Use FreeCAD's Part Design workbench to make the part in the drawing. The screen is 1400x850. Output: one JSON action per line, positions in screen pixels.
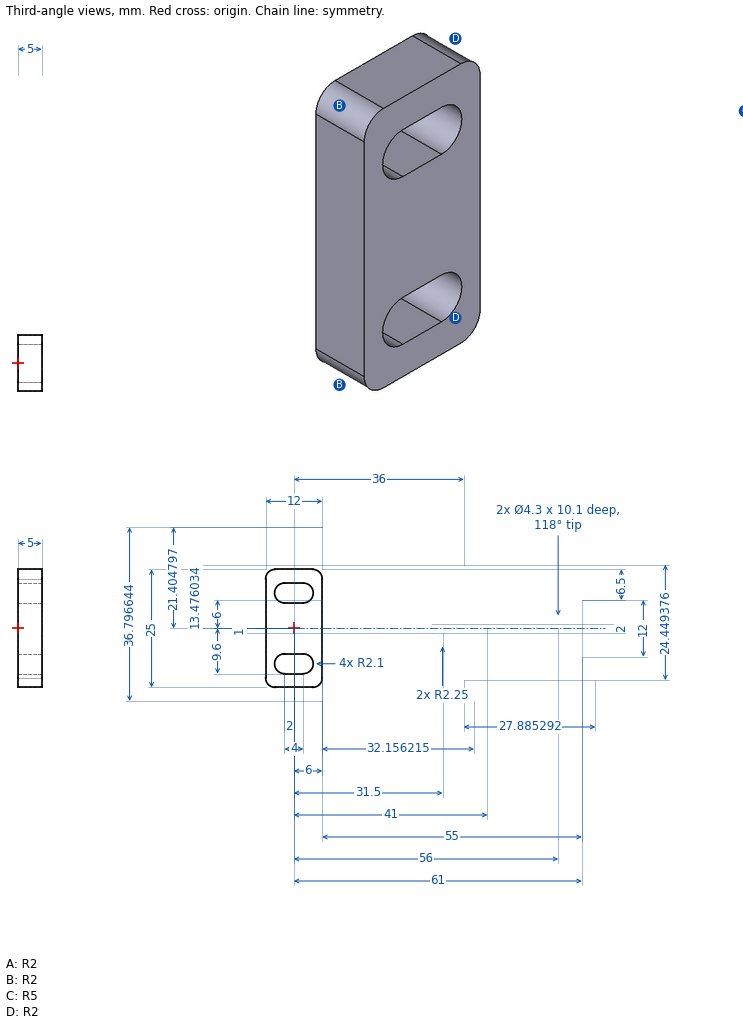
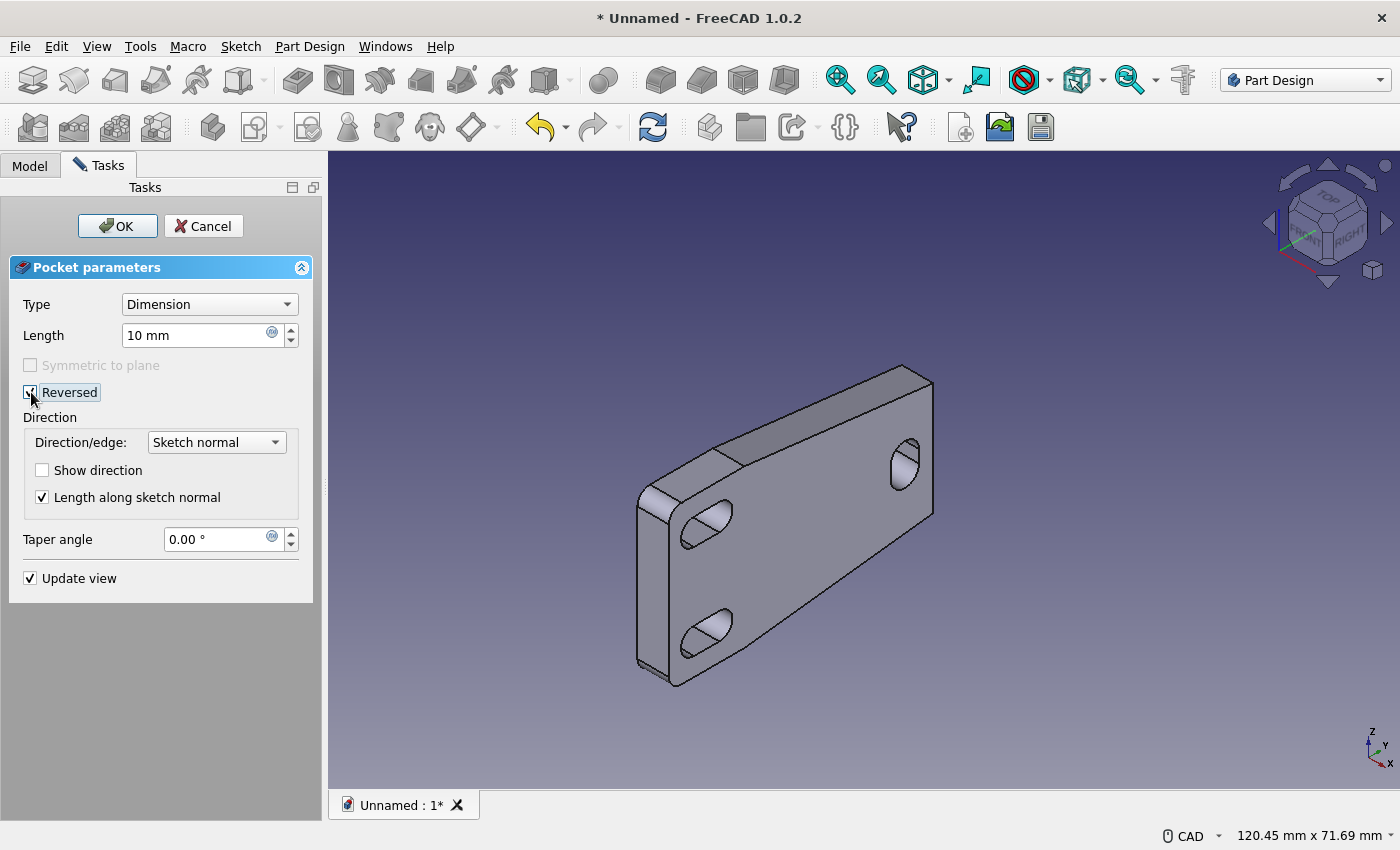
{"action": "left_click", "coordinate": [118, 226]}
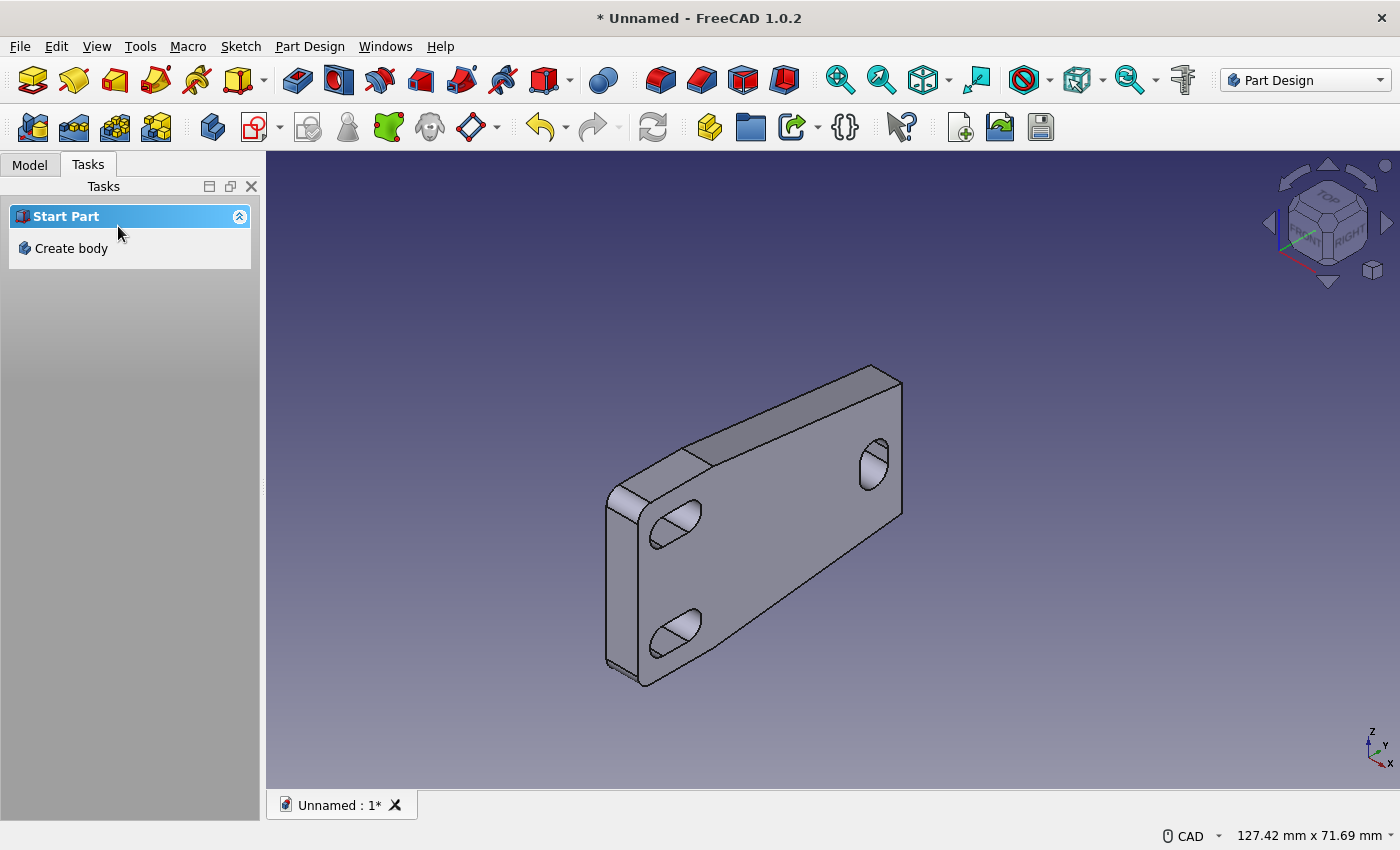
{"action": "key", "text": "2"}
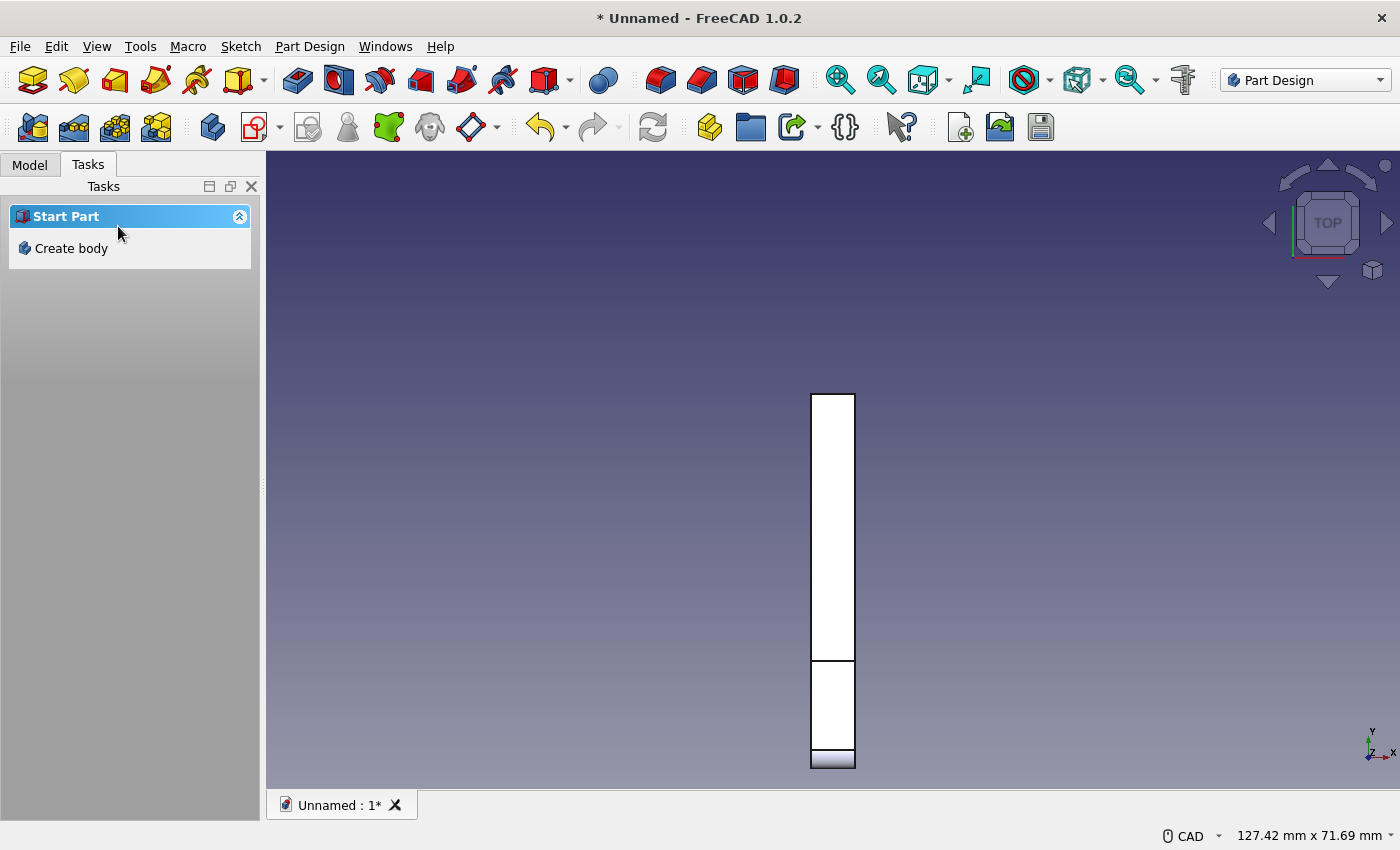
{"action": "key", "text": "0"}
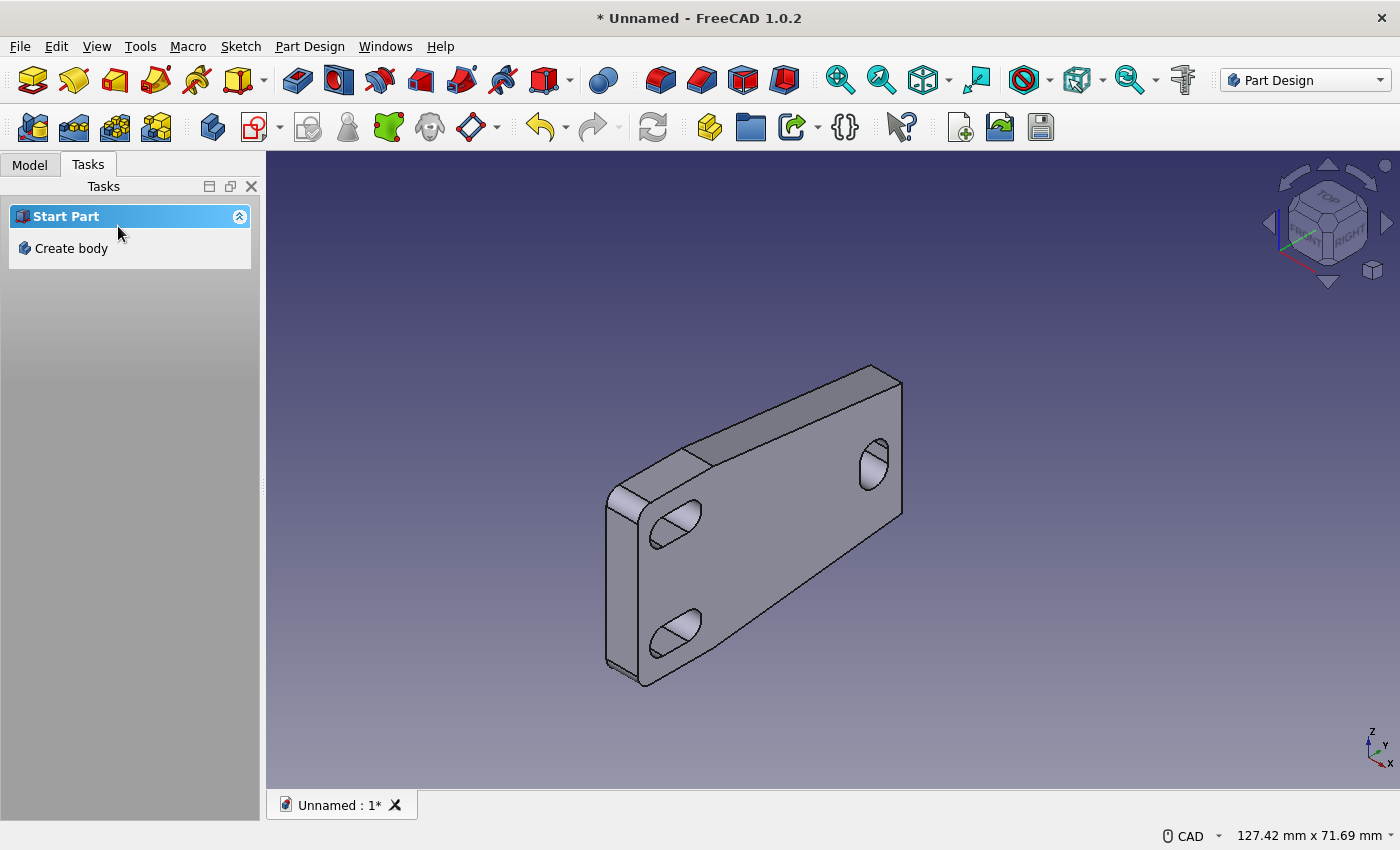
{"action": "key", "text": "1"}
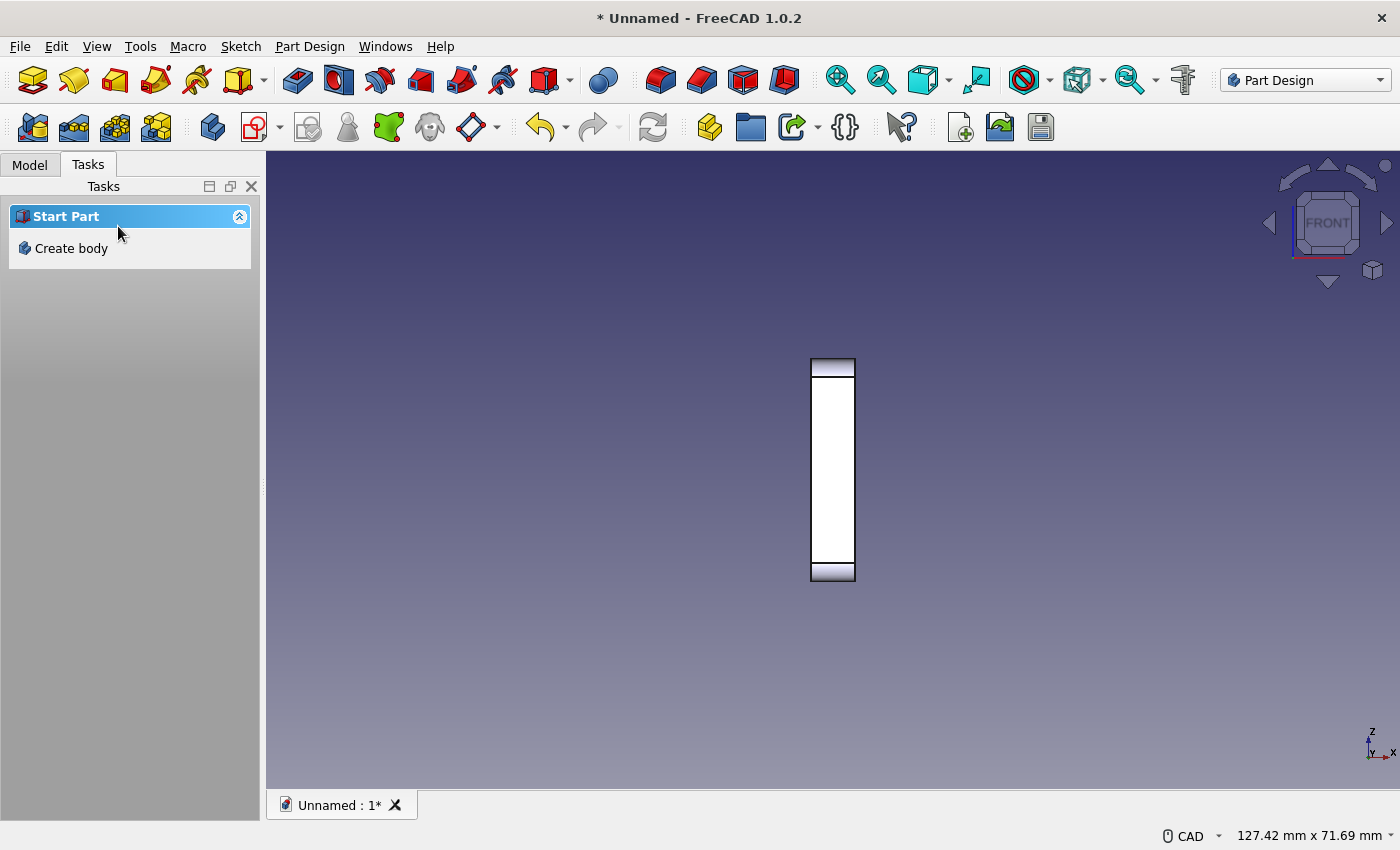
{"action": "left_click", "coordinate": [841, 80]}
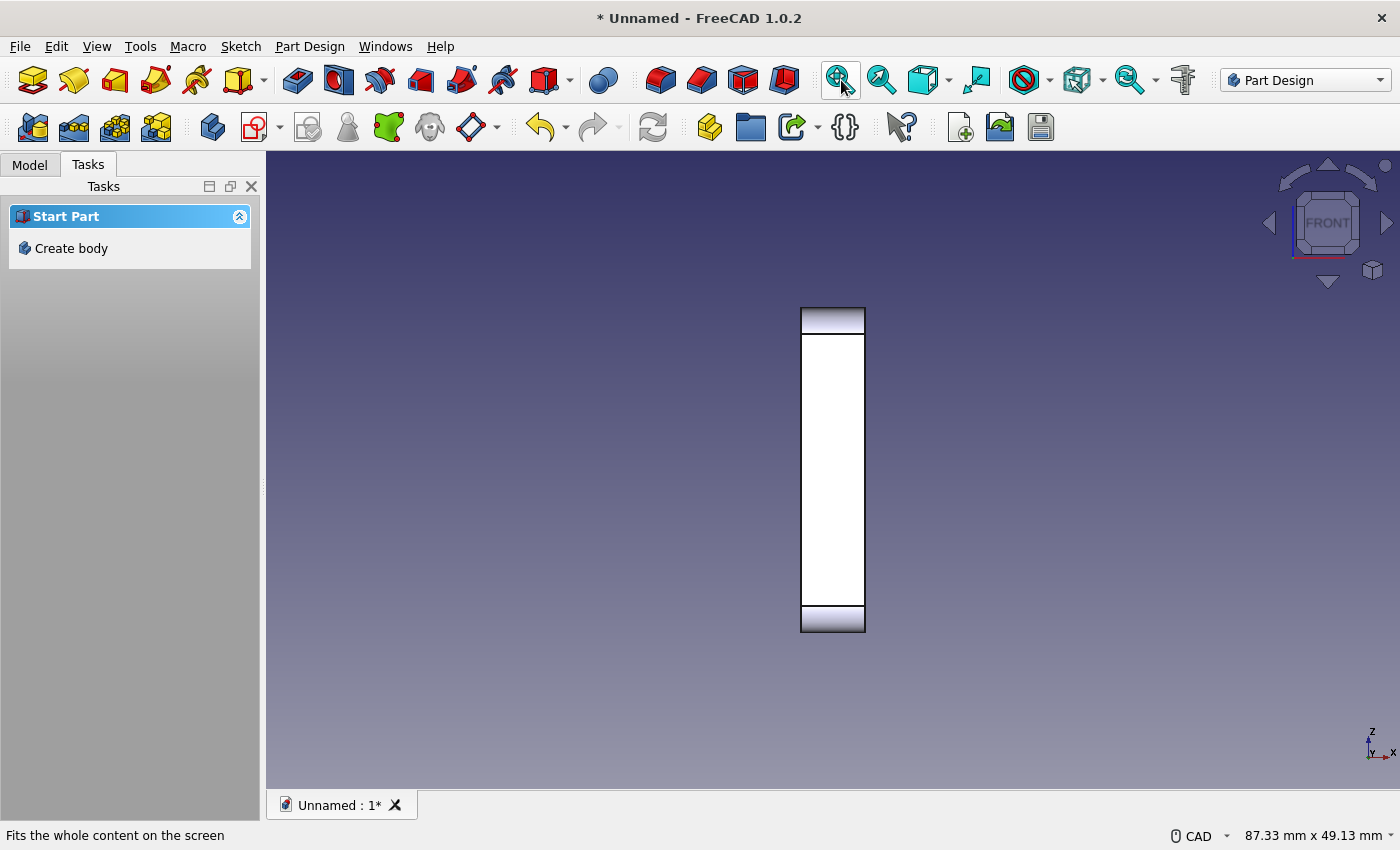
{"action": "key", "text": "3"}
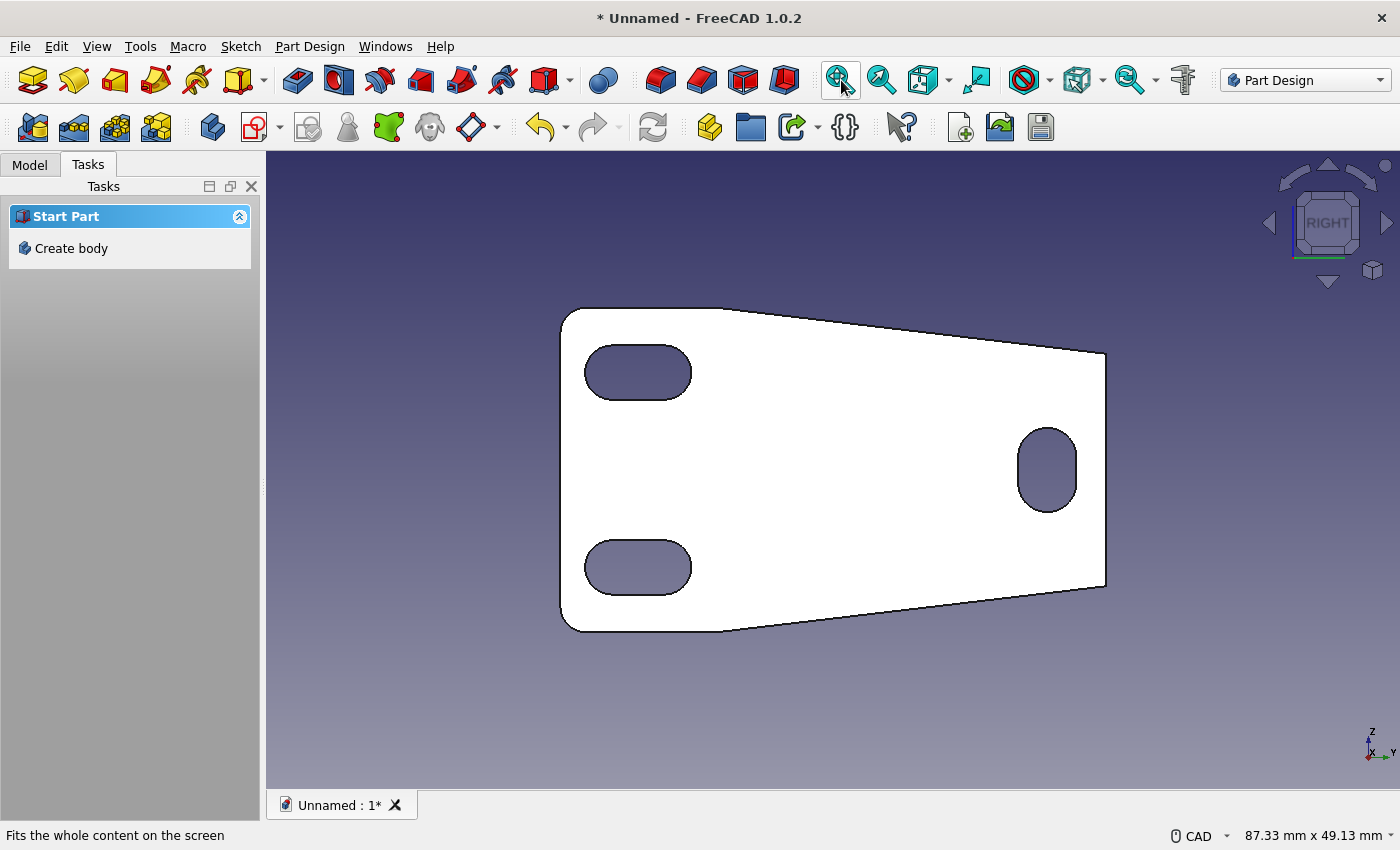
{"action": "key", "text": "5"}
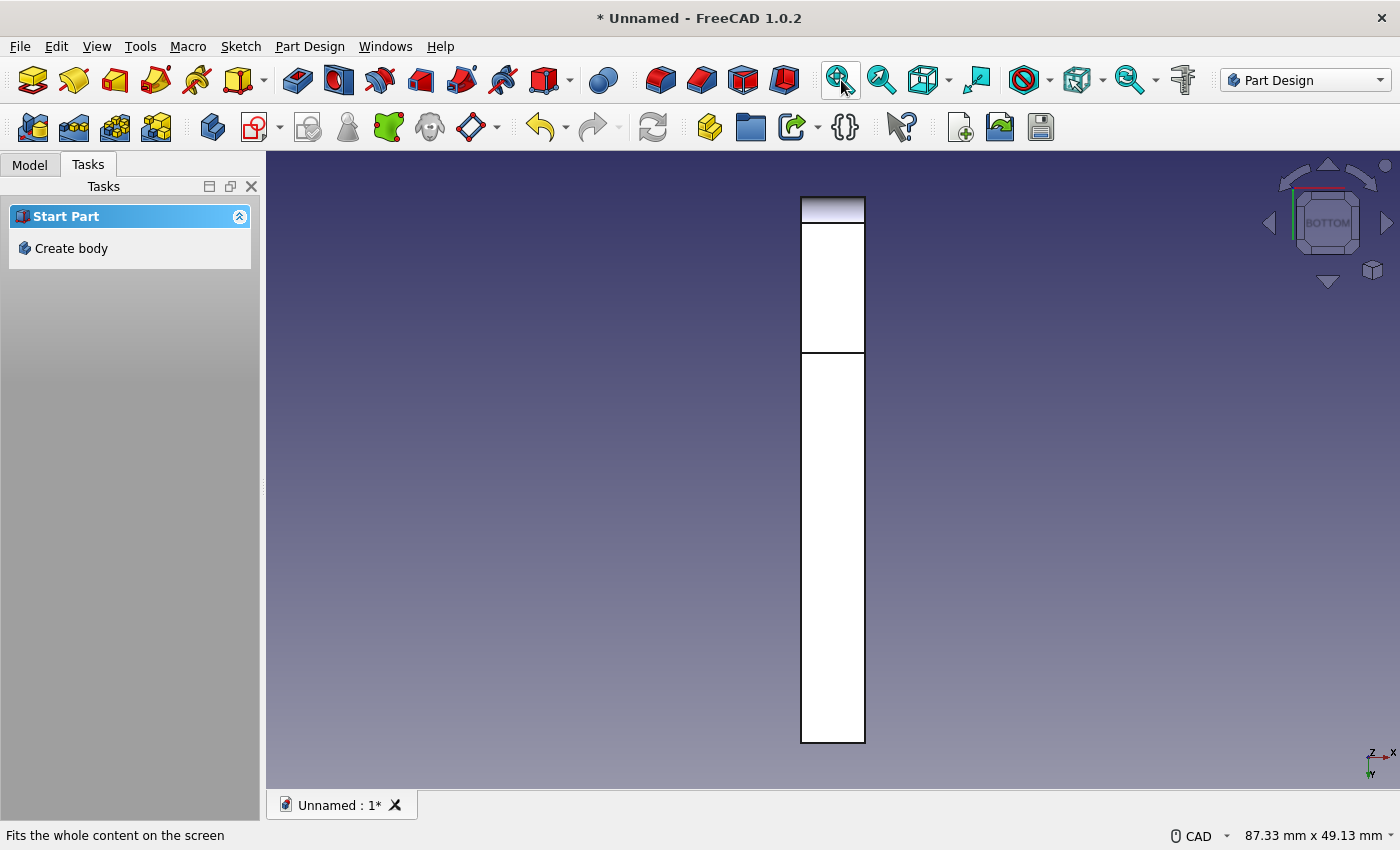
{"action": "key", "text": "4"}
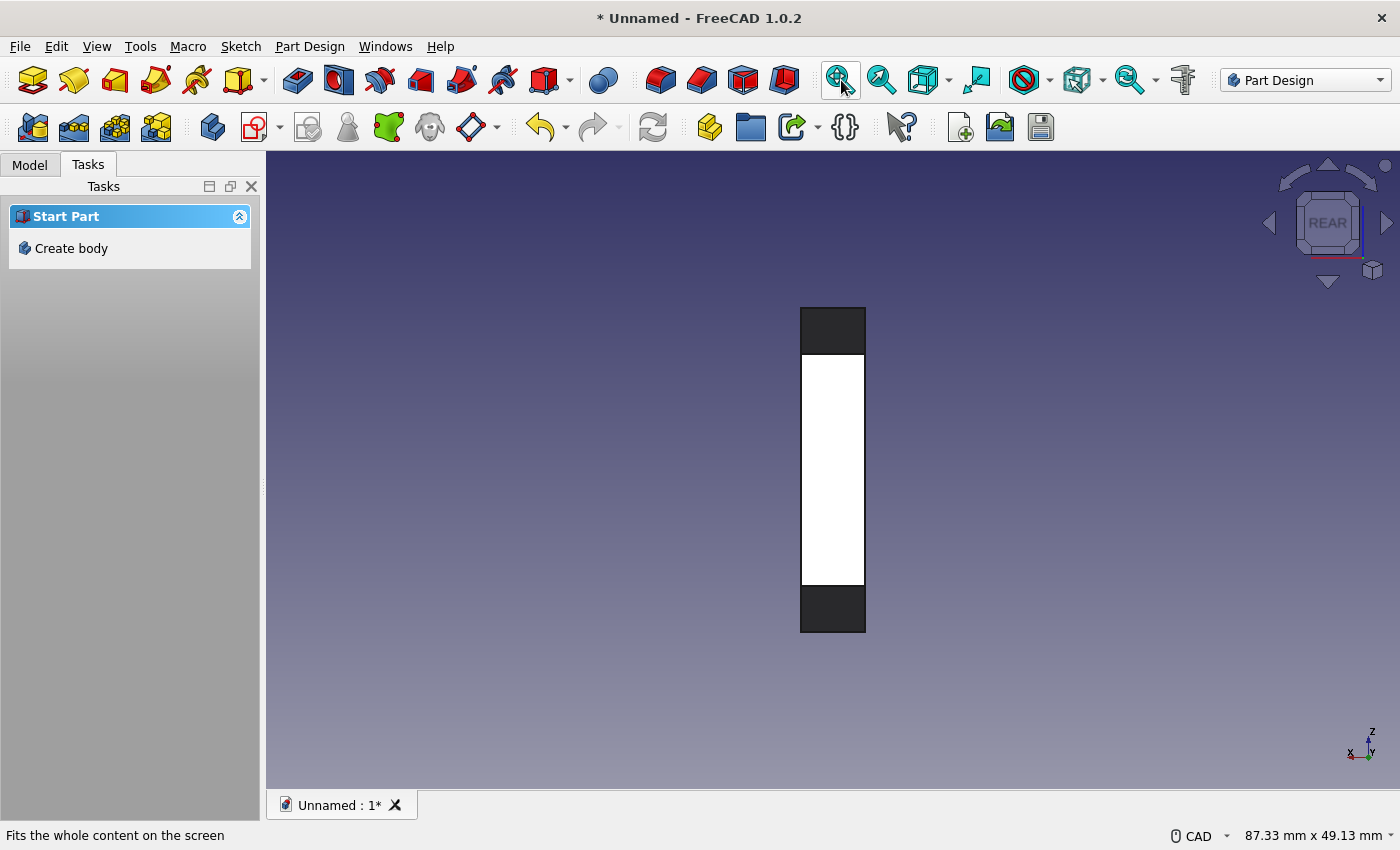
{"action": "left_click", "coordinate": [833, 353]}